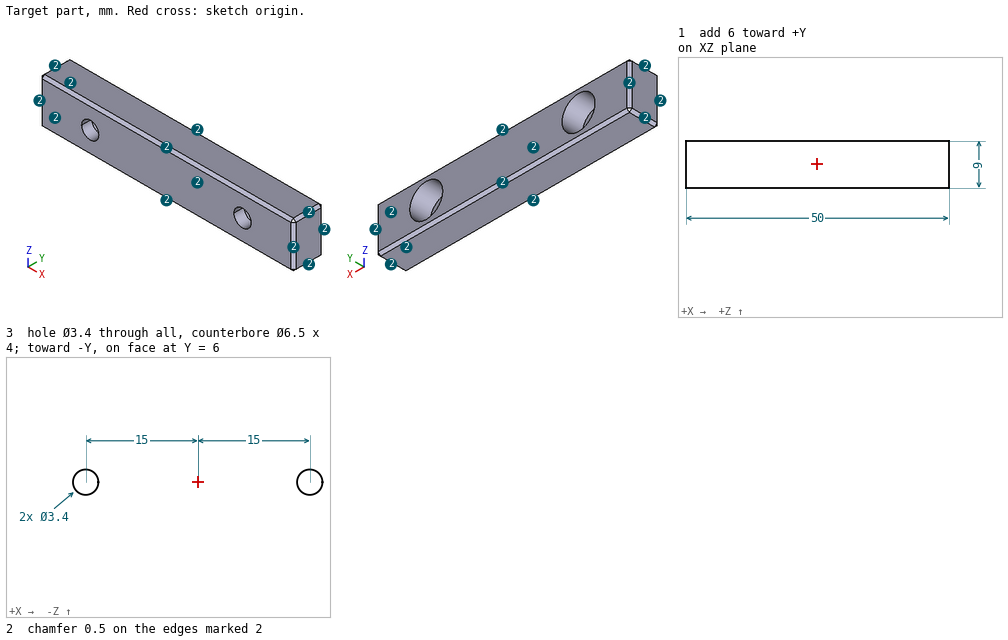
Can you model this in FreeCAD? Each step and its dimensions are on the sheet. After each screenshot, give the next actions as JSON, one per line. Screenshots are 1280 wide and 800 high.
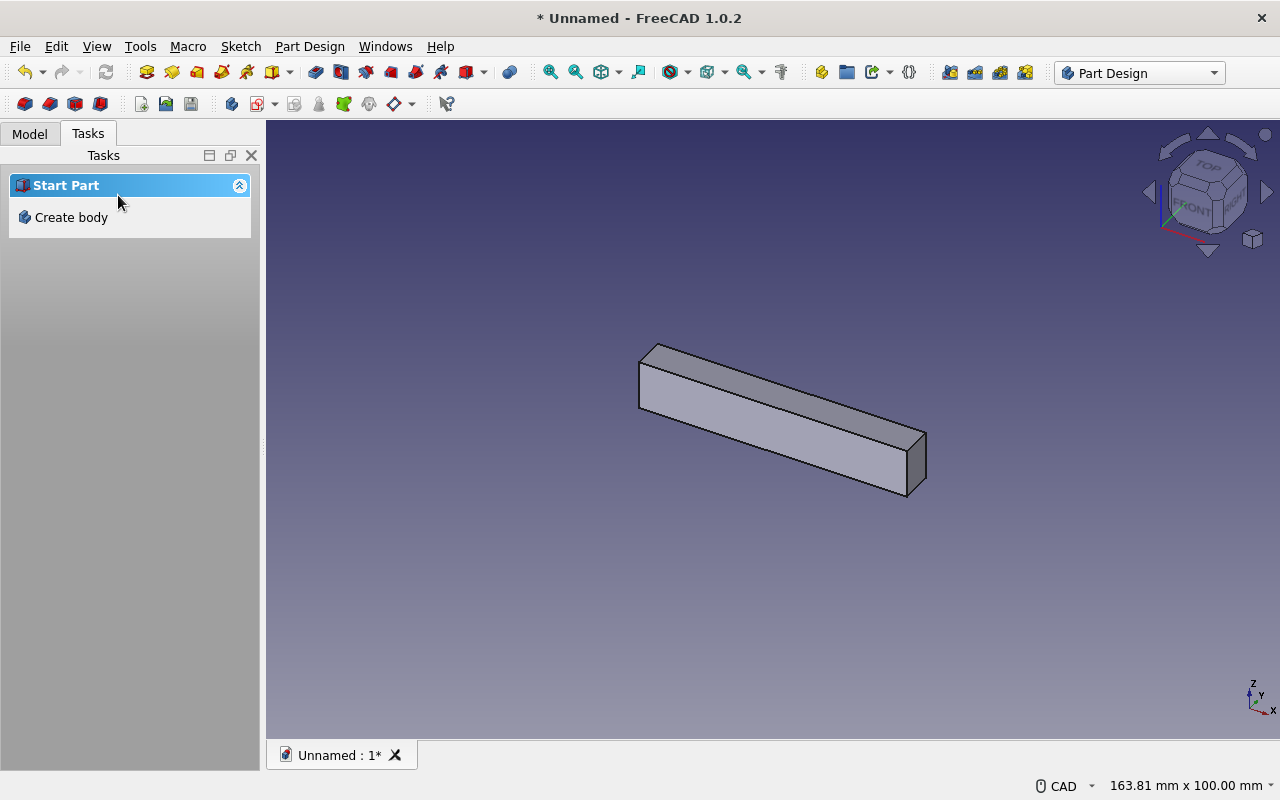
{"action": "left_click", "coordinate": [551, 72]}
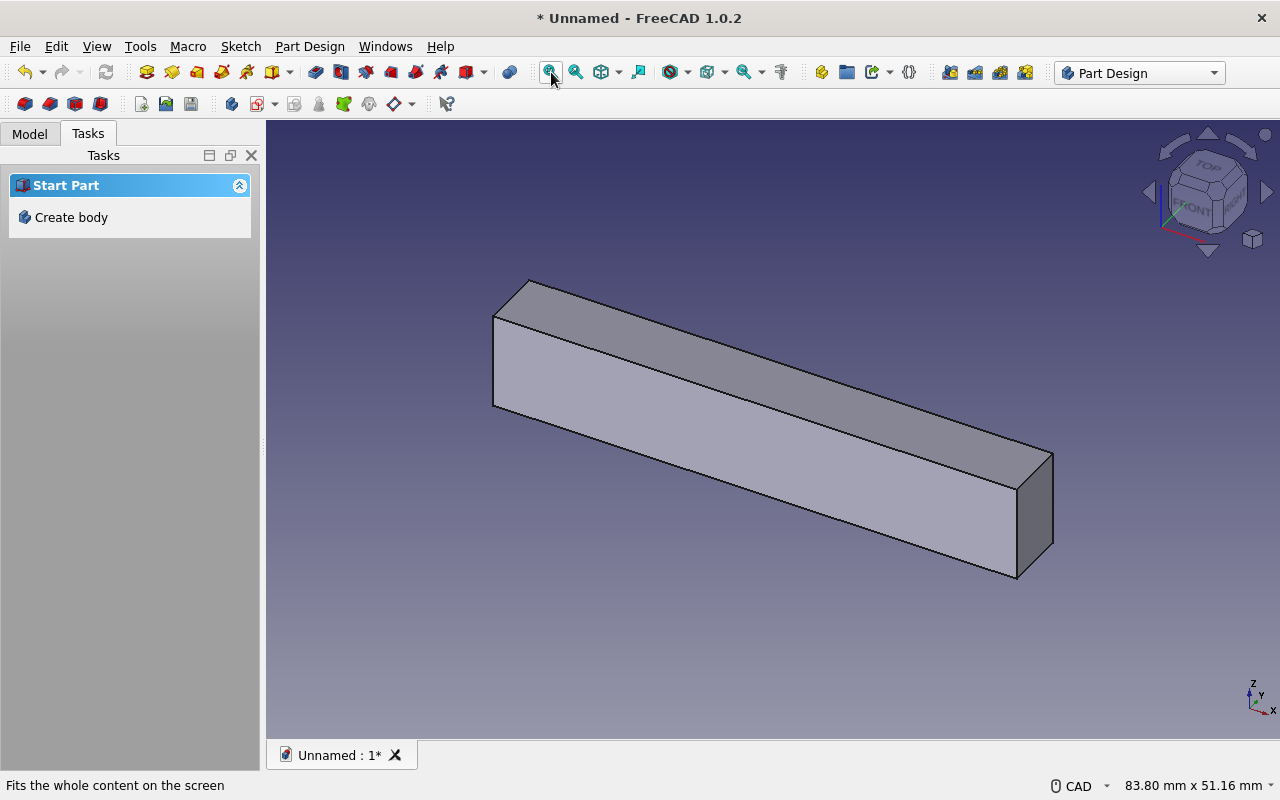
{"action": "left_click", "coordinate": [905, 496]}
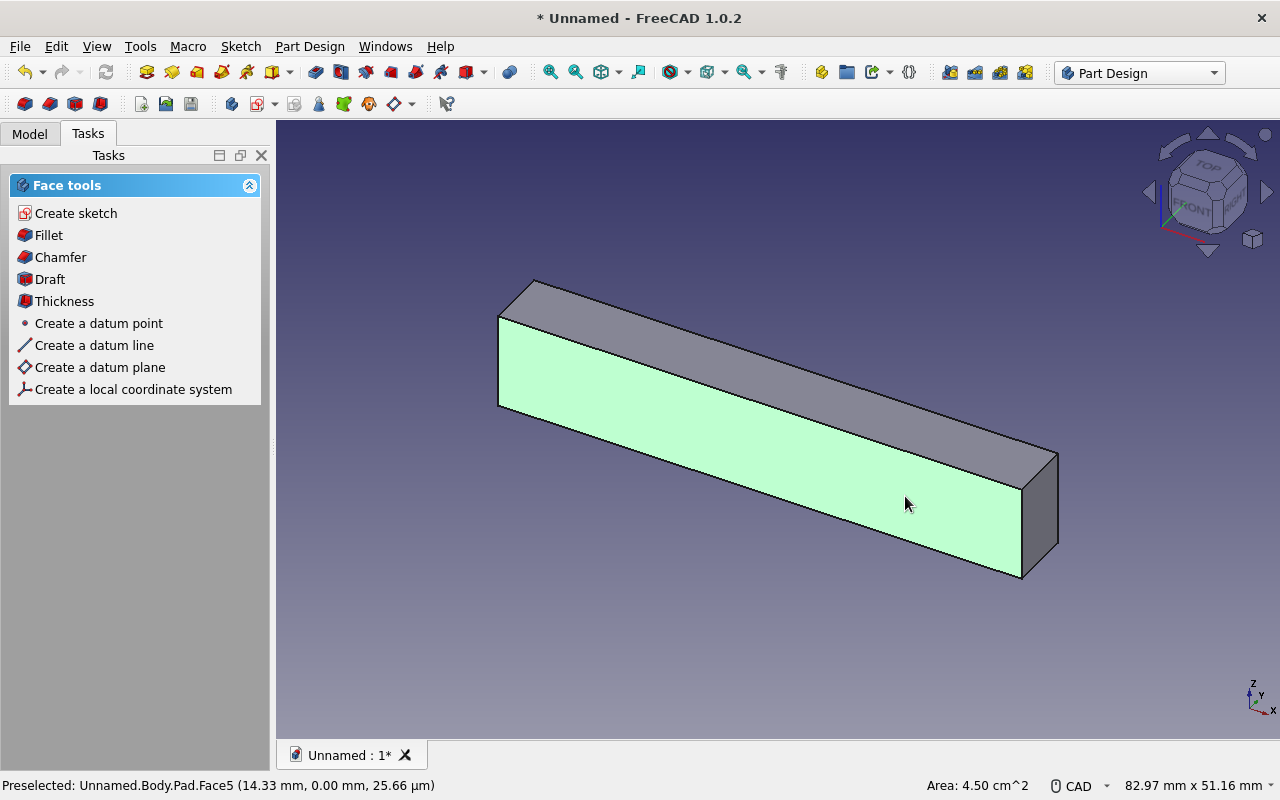
{"action": "left_click", "coordinate": [1040, 471], "text": "ctrl"}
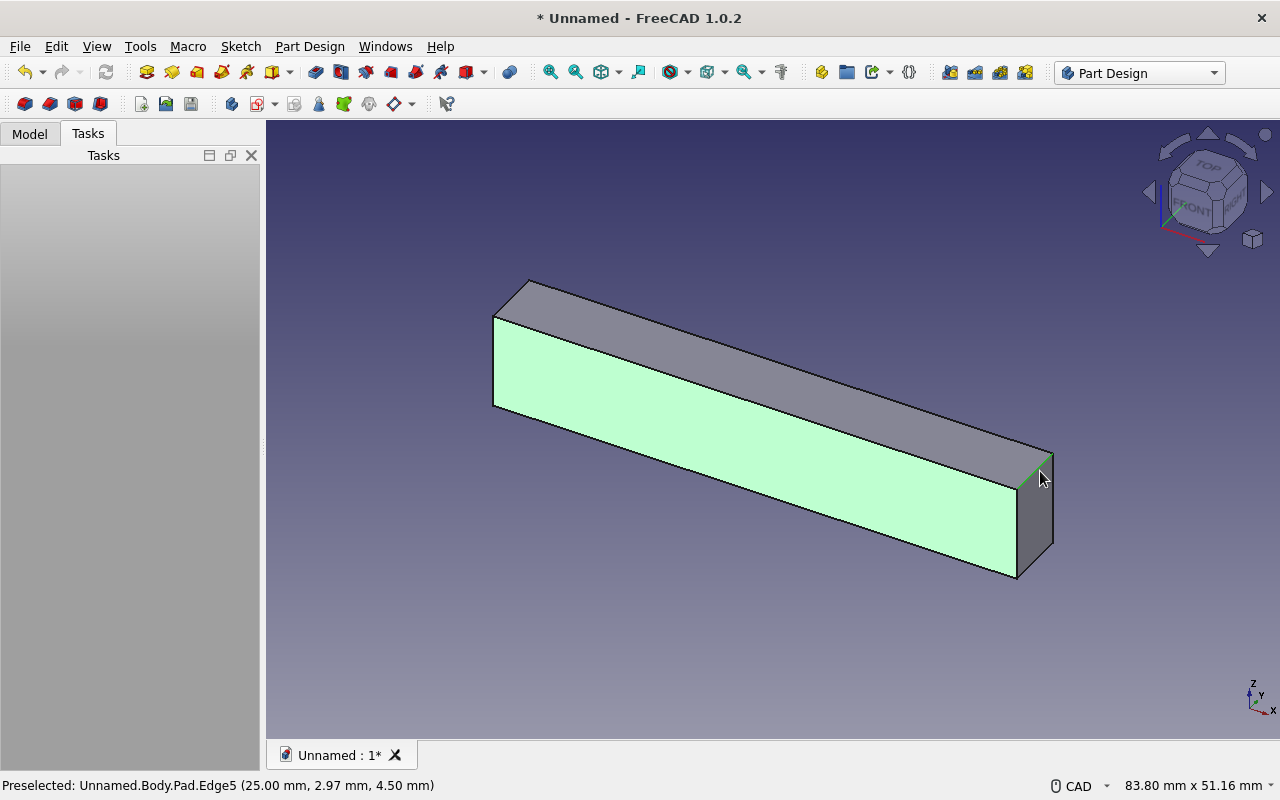
{"action": "key", "text": "0"}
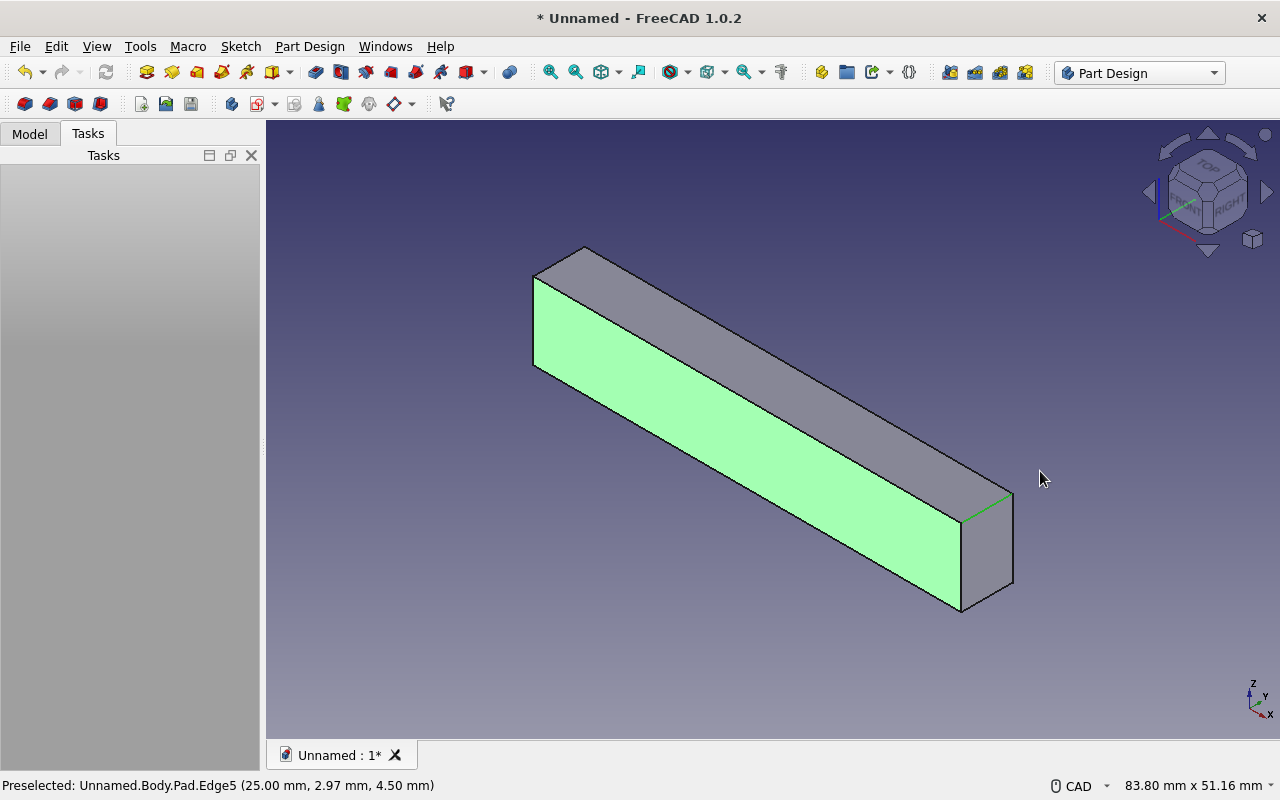
{"action": "key", "text": "2"}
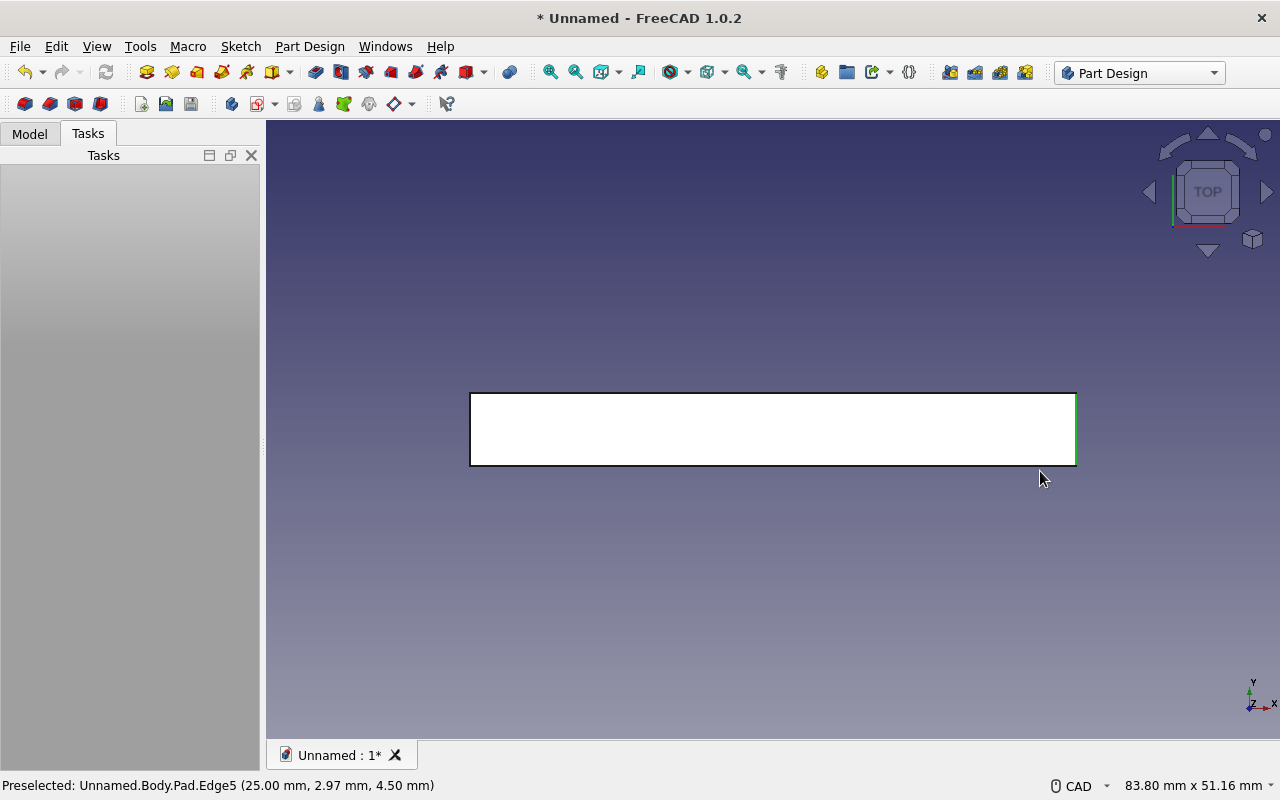
{"action": "left_click", "coordinate": [470, 429], "text": "ctrl"}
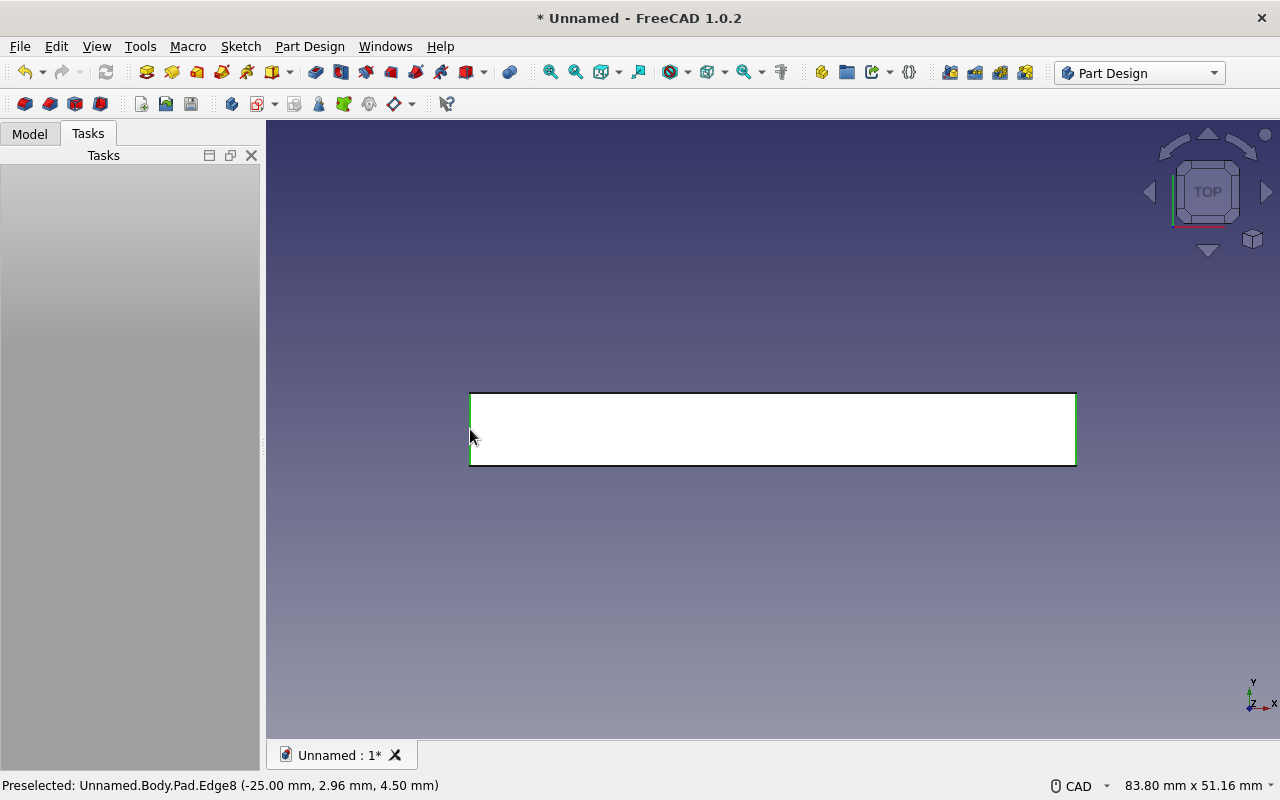
{"action": "key", "text": "1"}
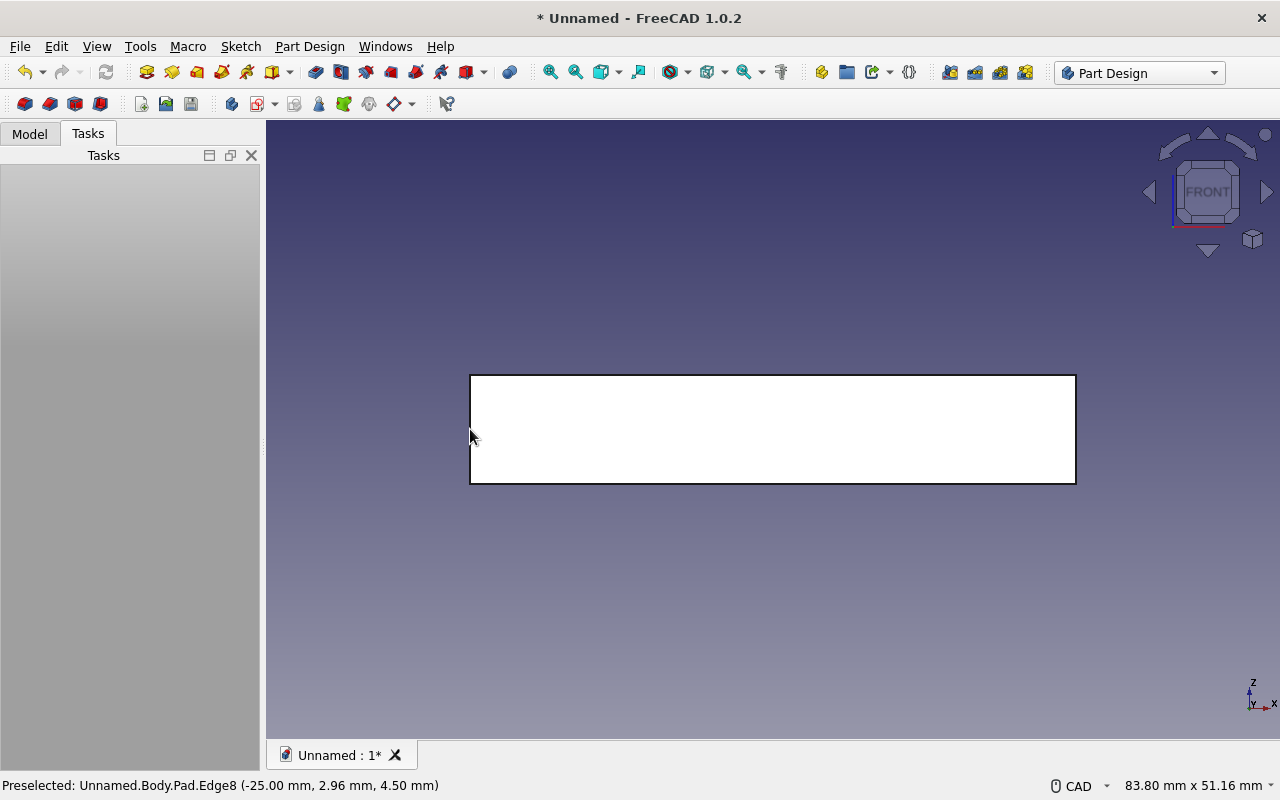
{"action": "key", "text": "3"}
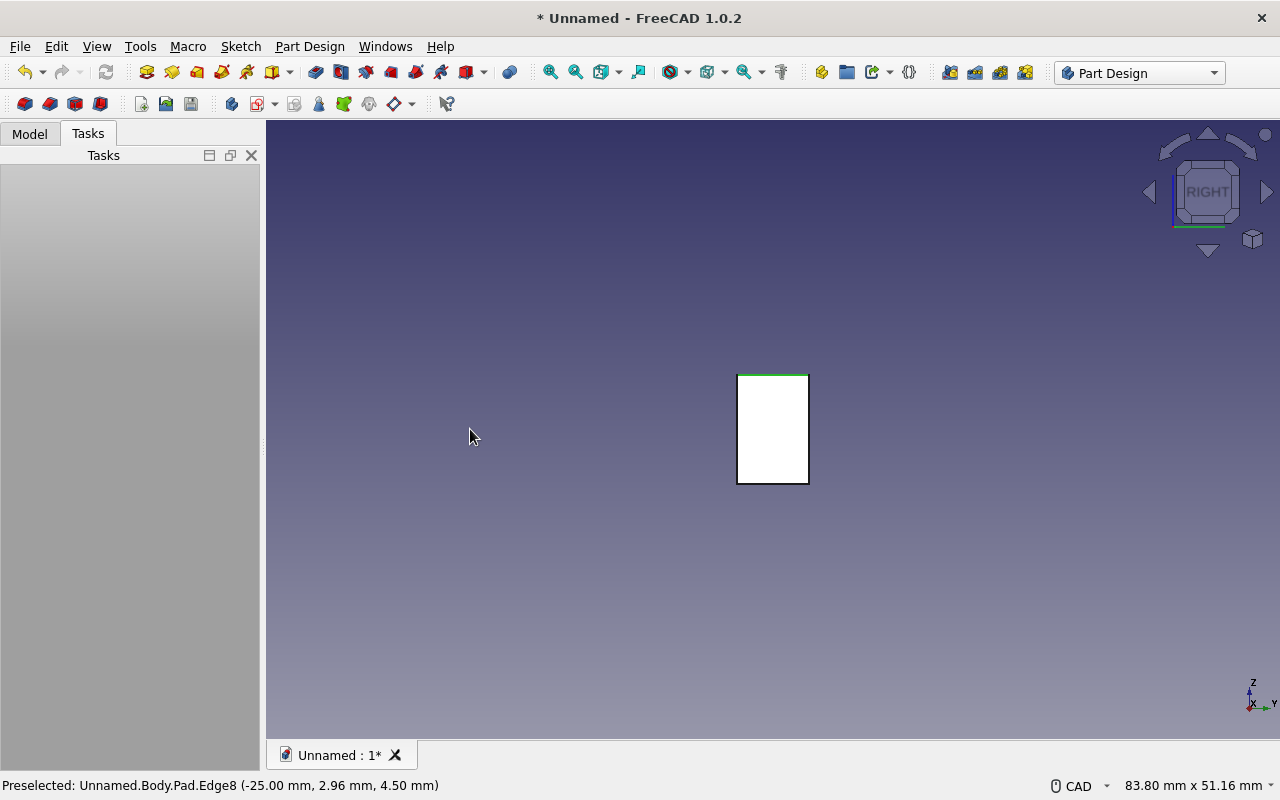
{"action": "left_click", "coordinate": [551, 72]}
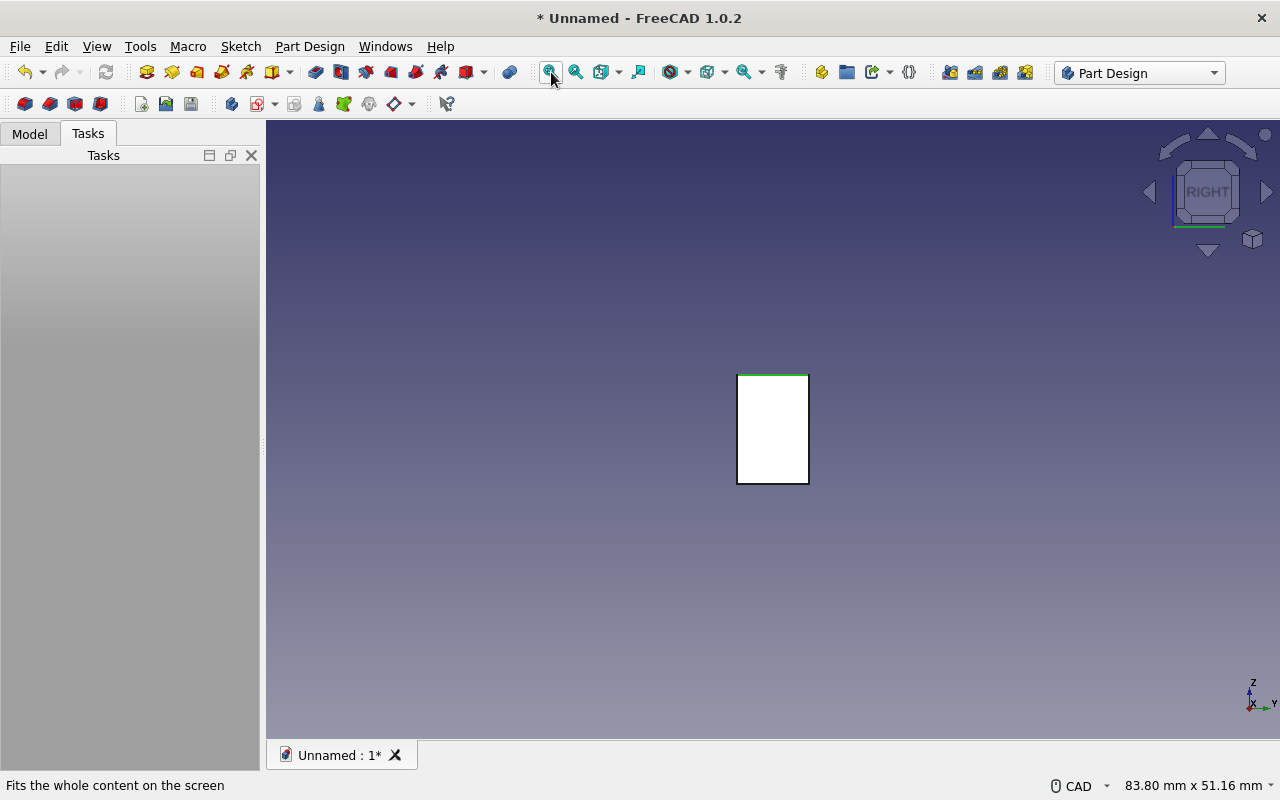
{"action": "left_click", "coordinate": [773, 483], "text": "ctrl"}